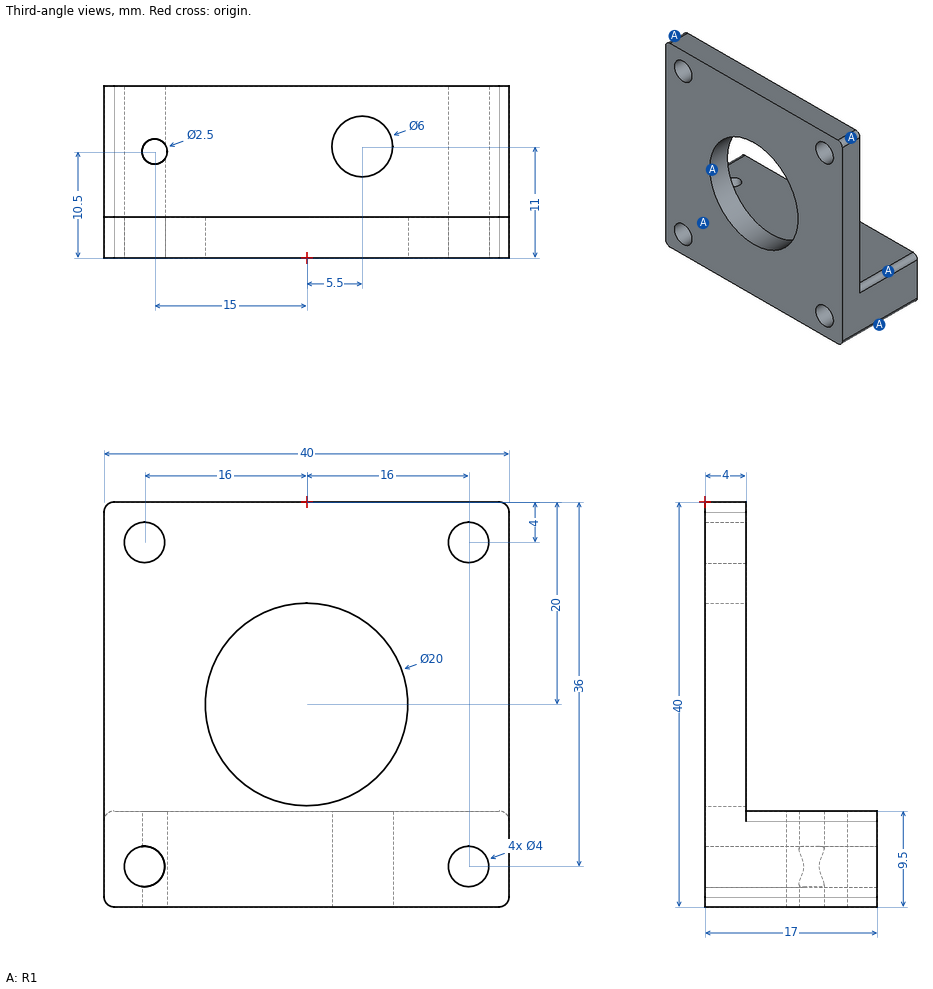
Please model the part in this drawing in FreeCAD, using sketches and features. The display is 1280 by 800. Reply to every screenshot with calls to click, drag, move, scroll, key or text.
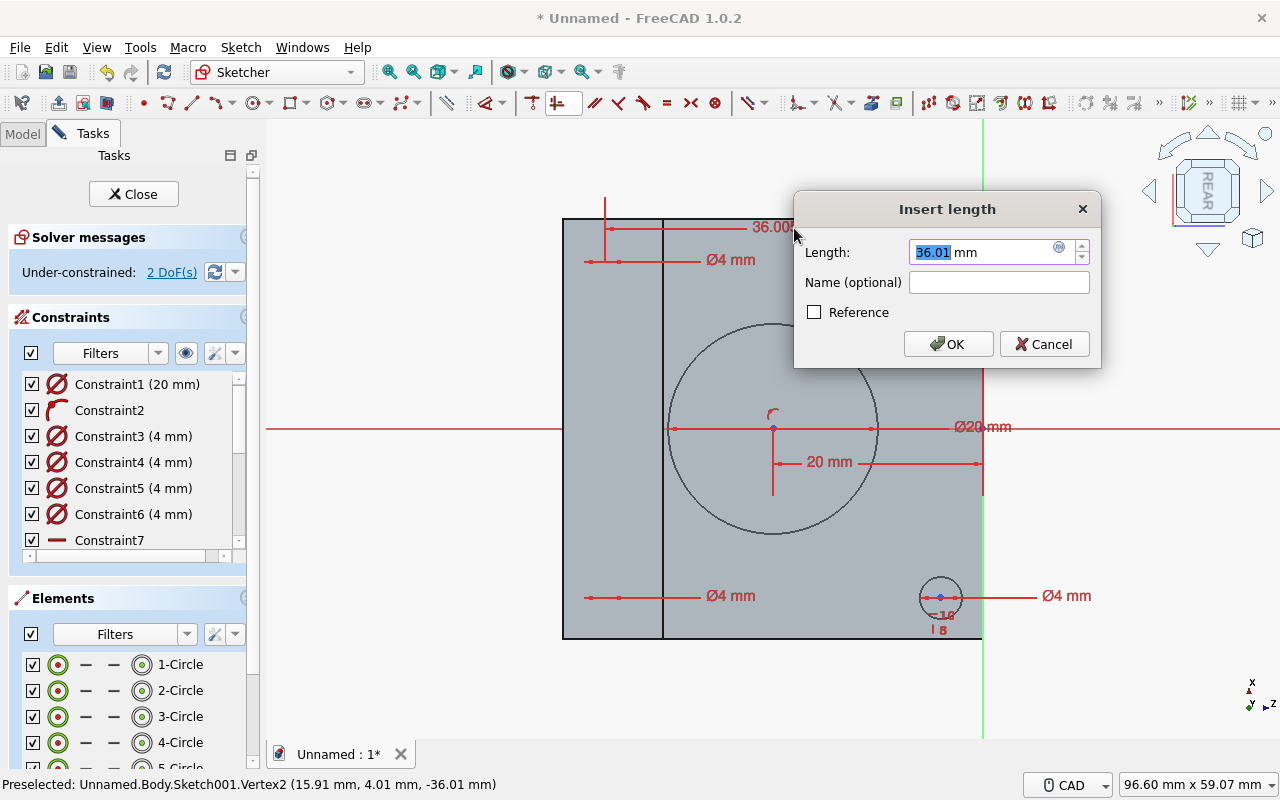
text(36)
key(Return)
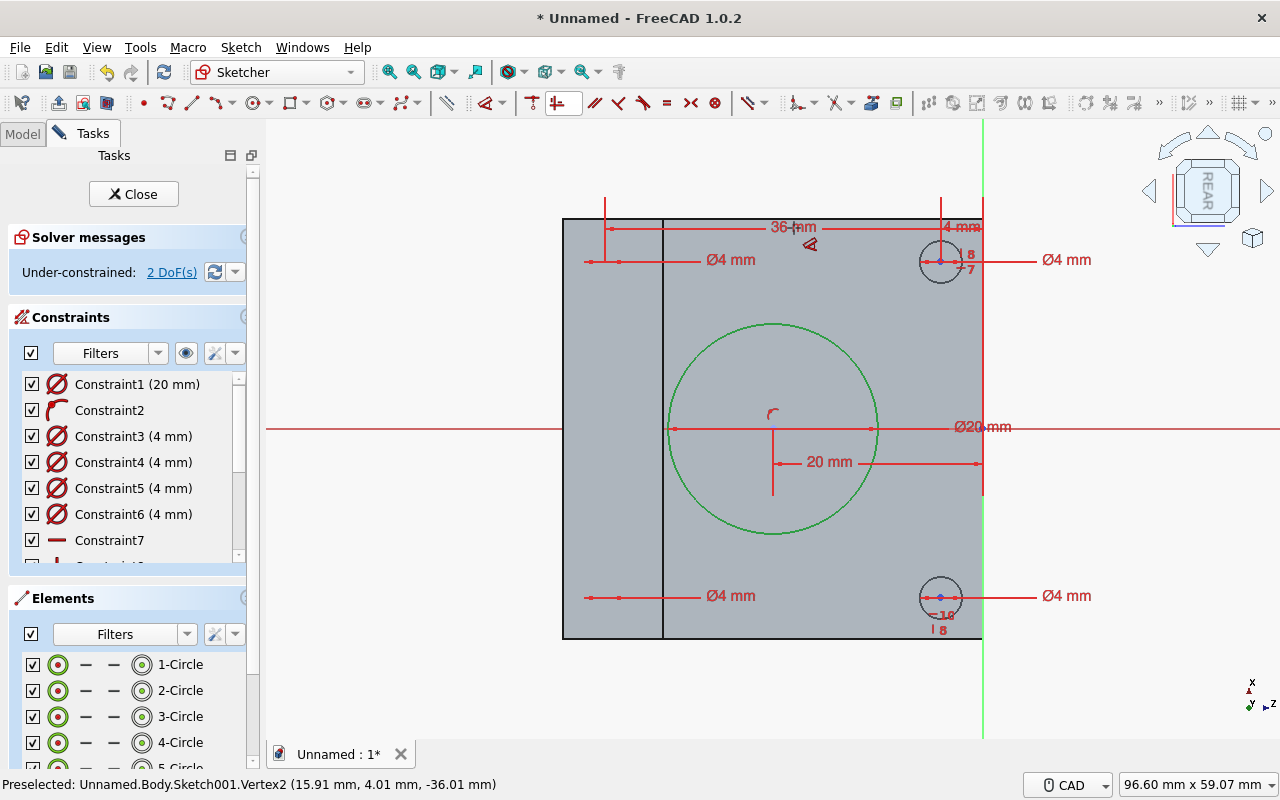
click(605, 262)
click(1017, 346)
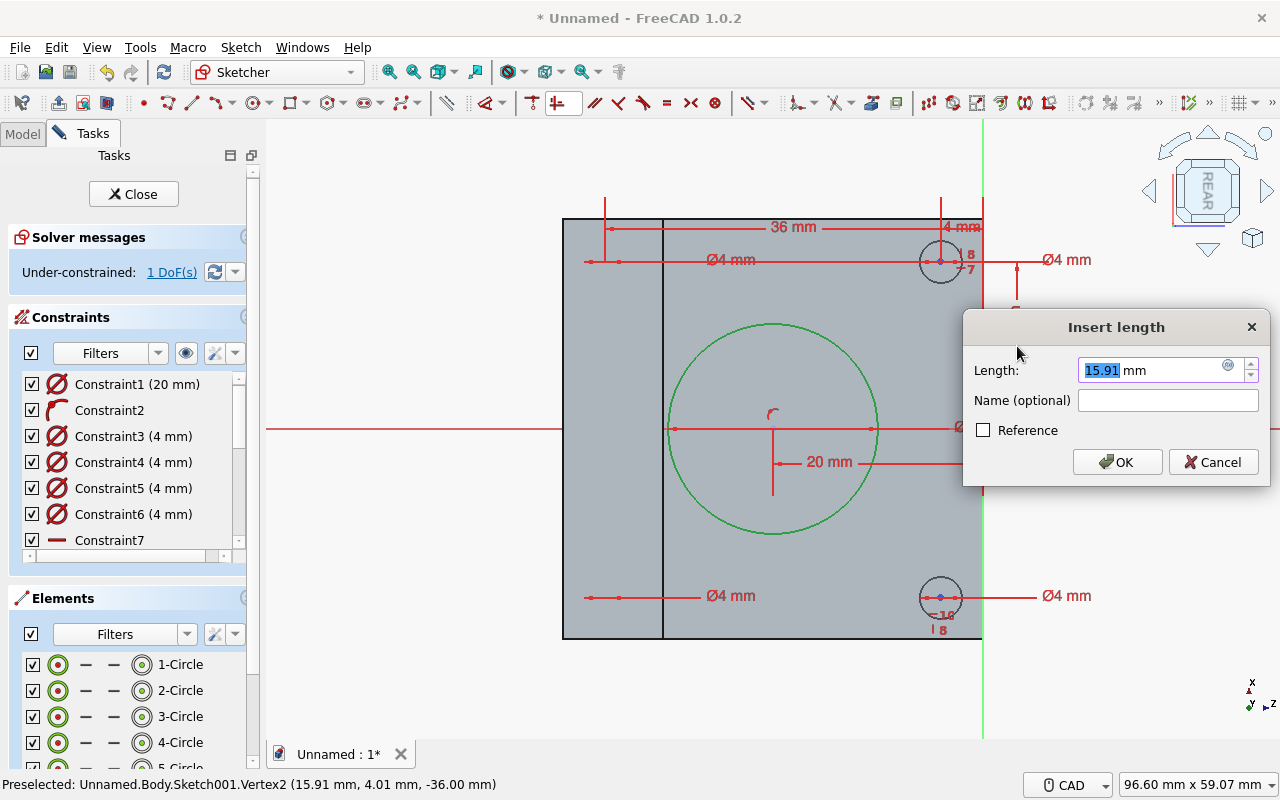
text(16)
key(Return)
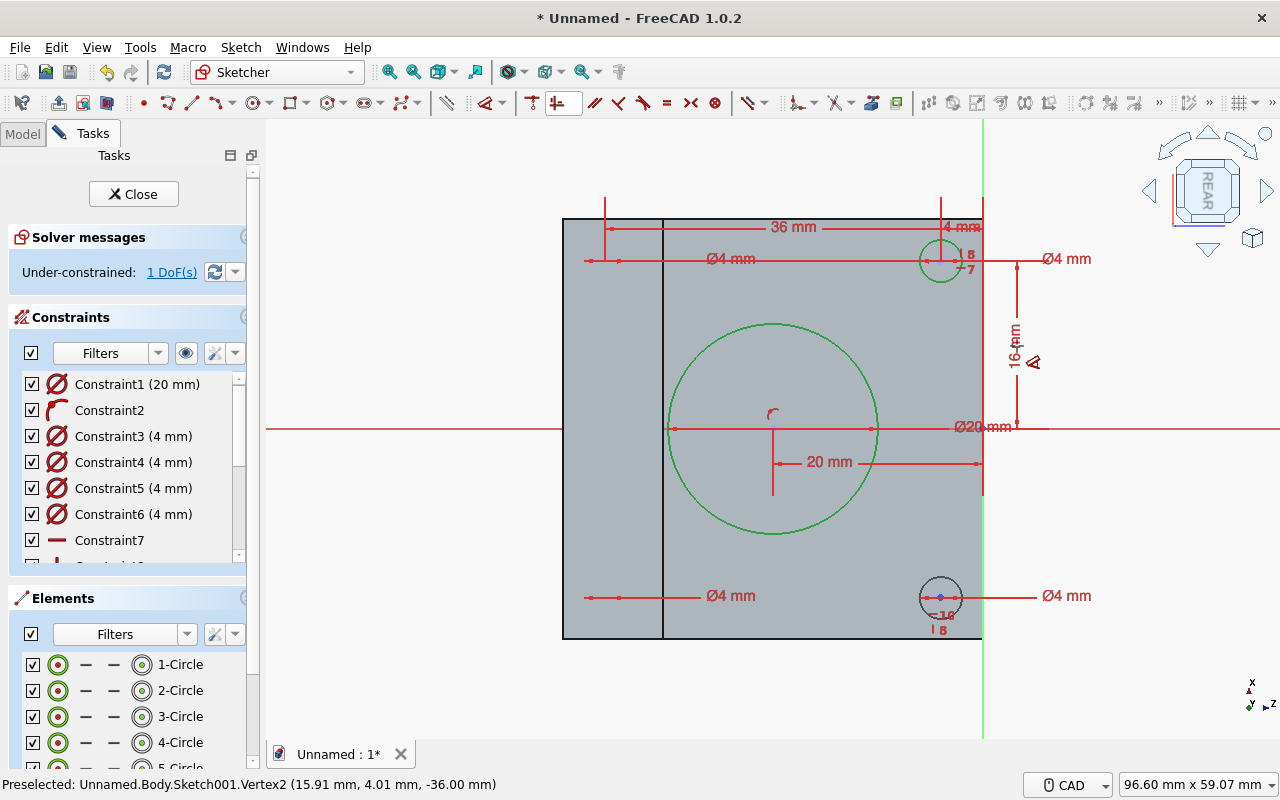
click(941, 598)
click(1017, 513)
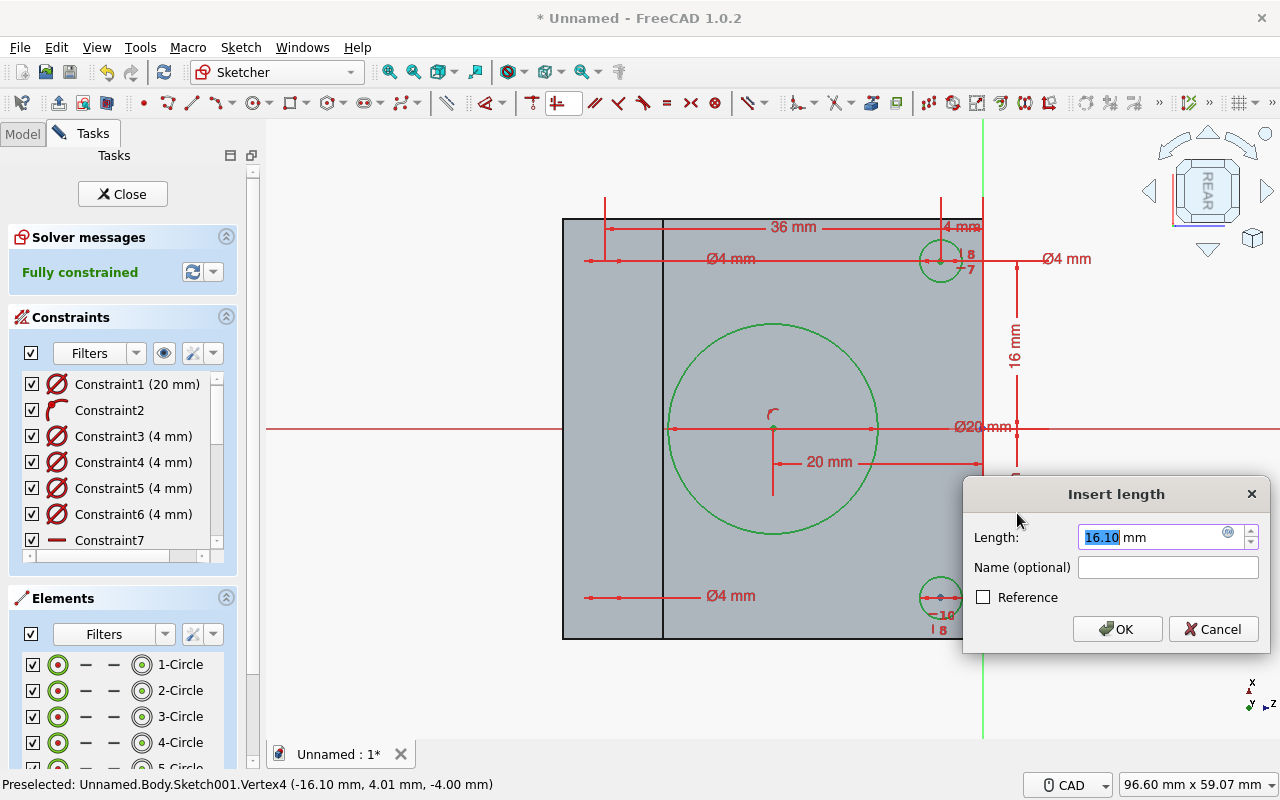
text(16)
key(Return)
key(Escape)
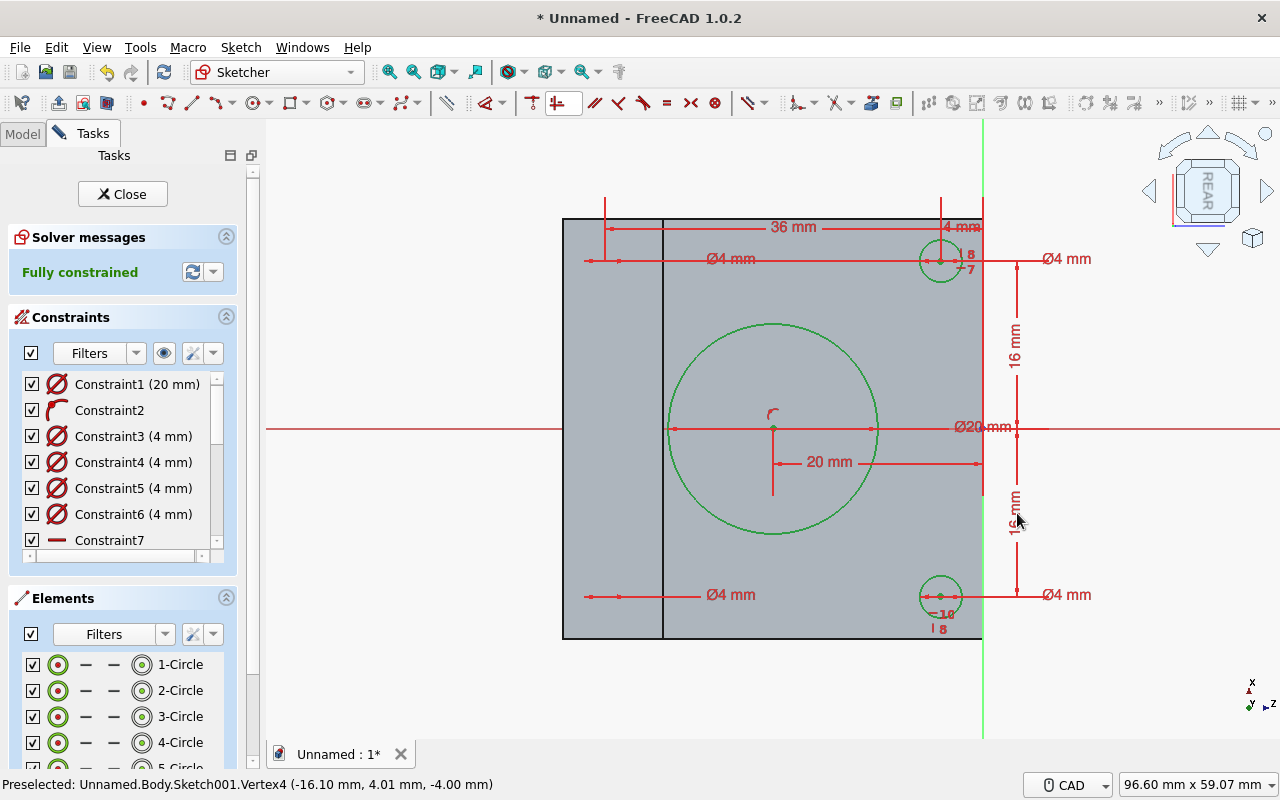
click(123, 194)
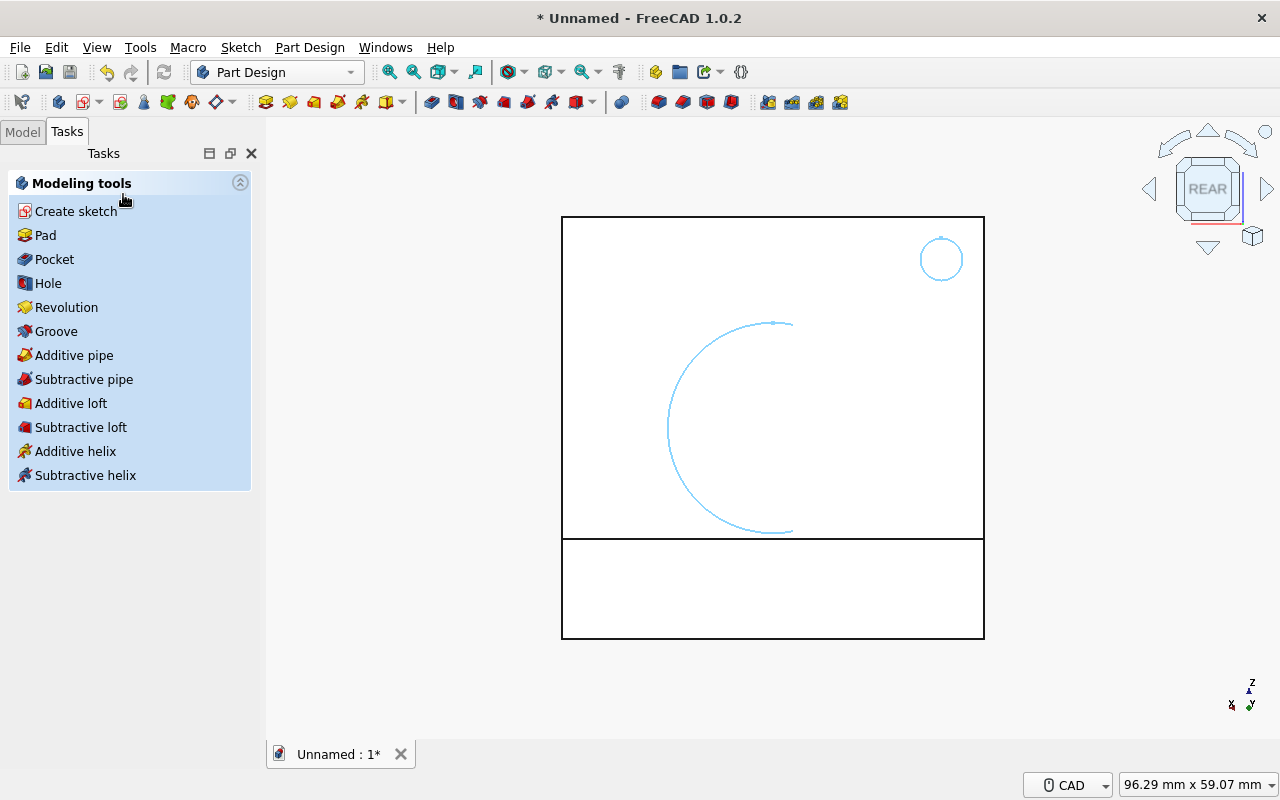
click(432, 102)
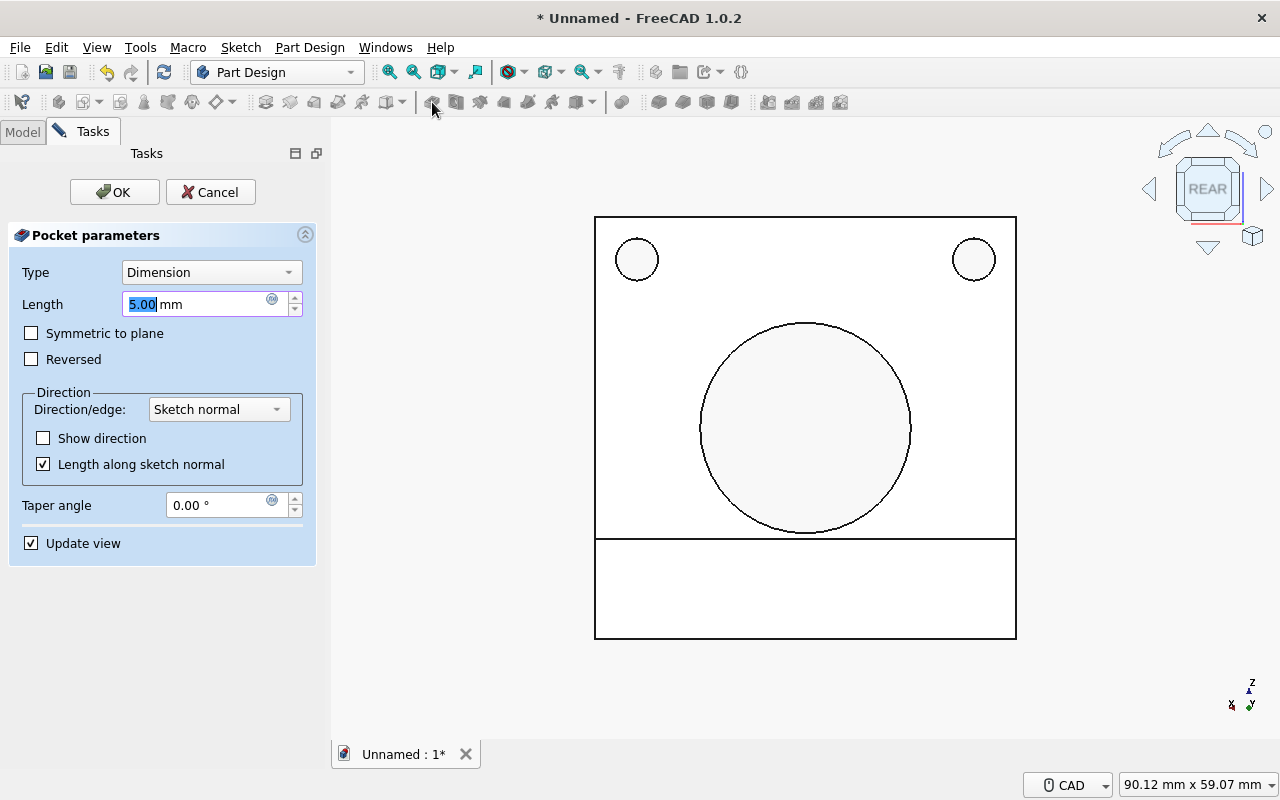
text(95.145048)
key(Tab)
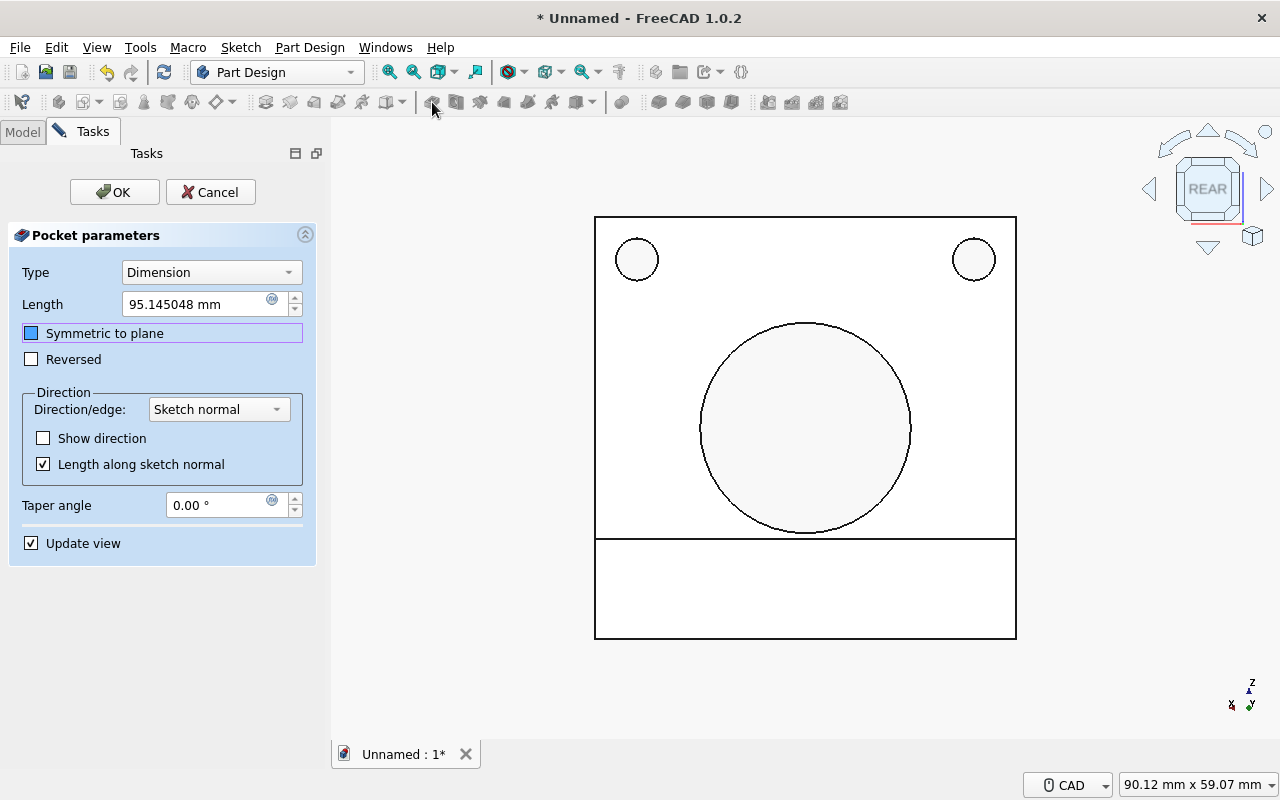
click(30, 333)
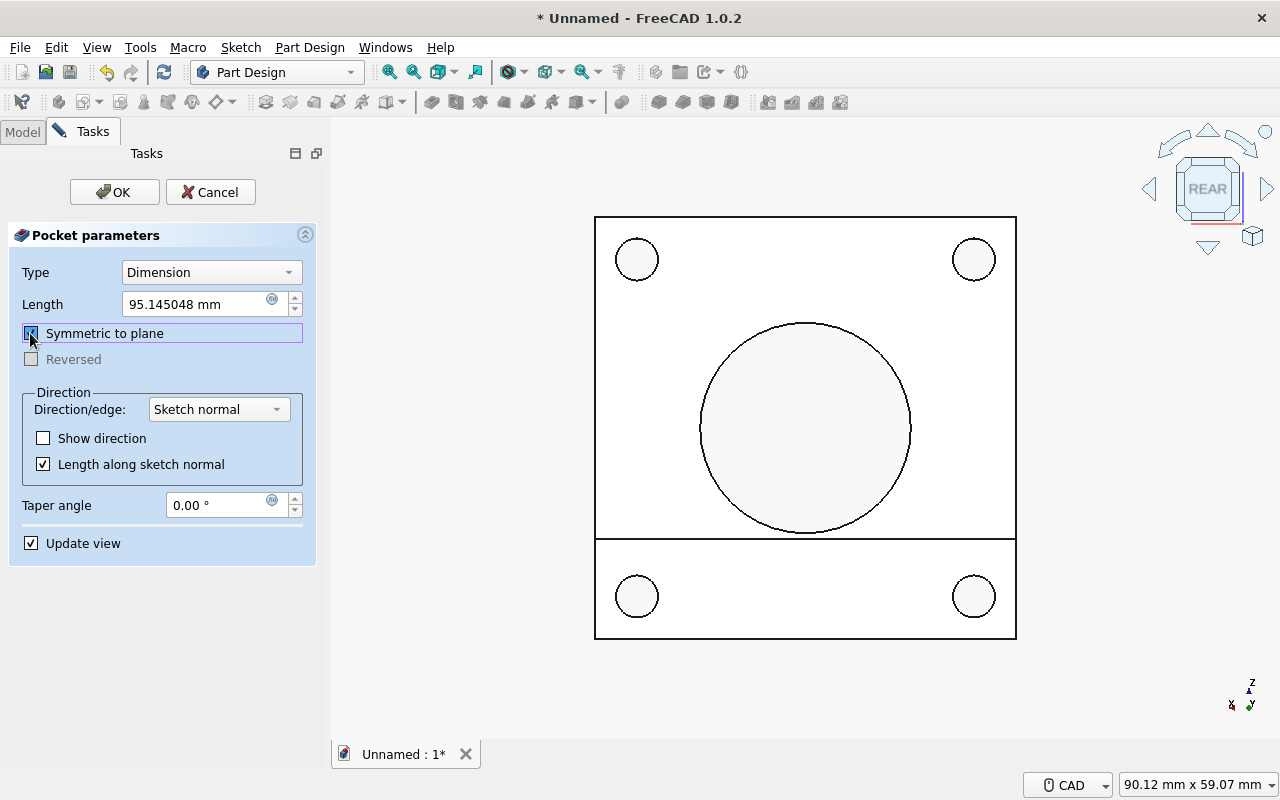
click(115, 192)